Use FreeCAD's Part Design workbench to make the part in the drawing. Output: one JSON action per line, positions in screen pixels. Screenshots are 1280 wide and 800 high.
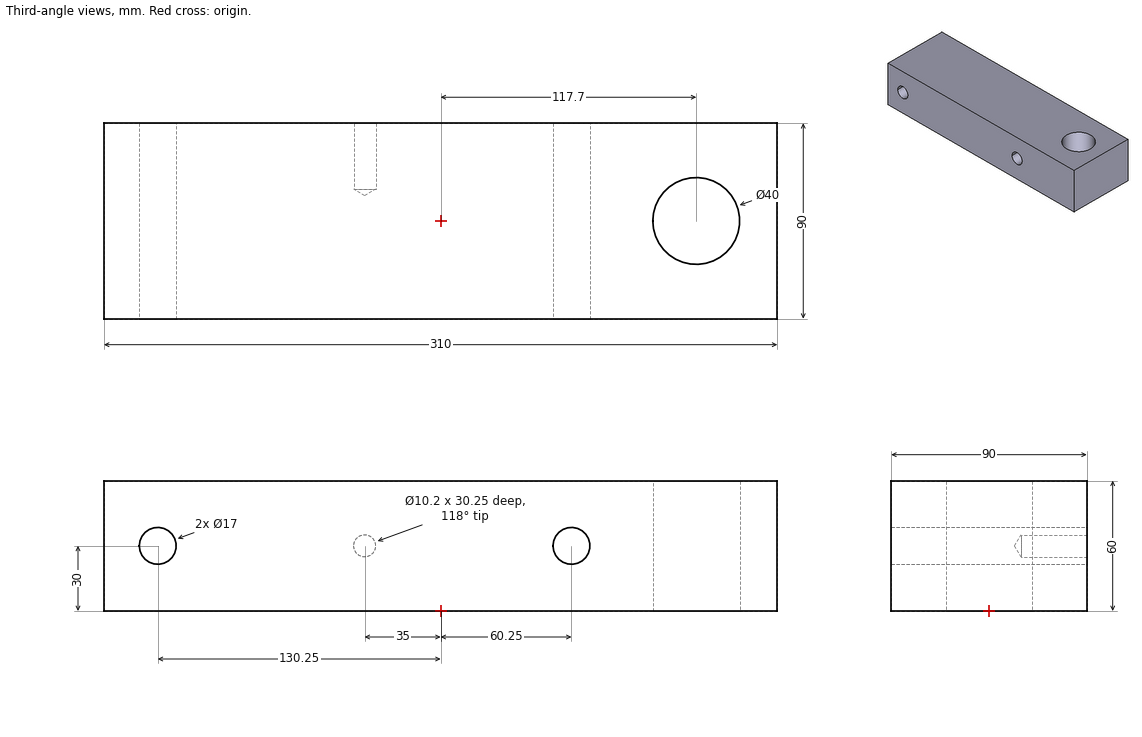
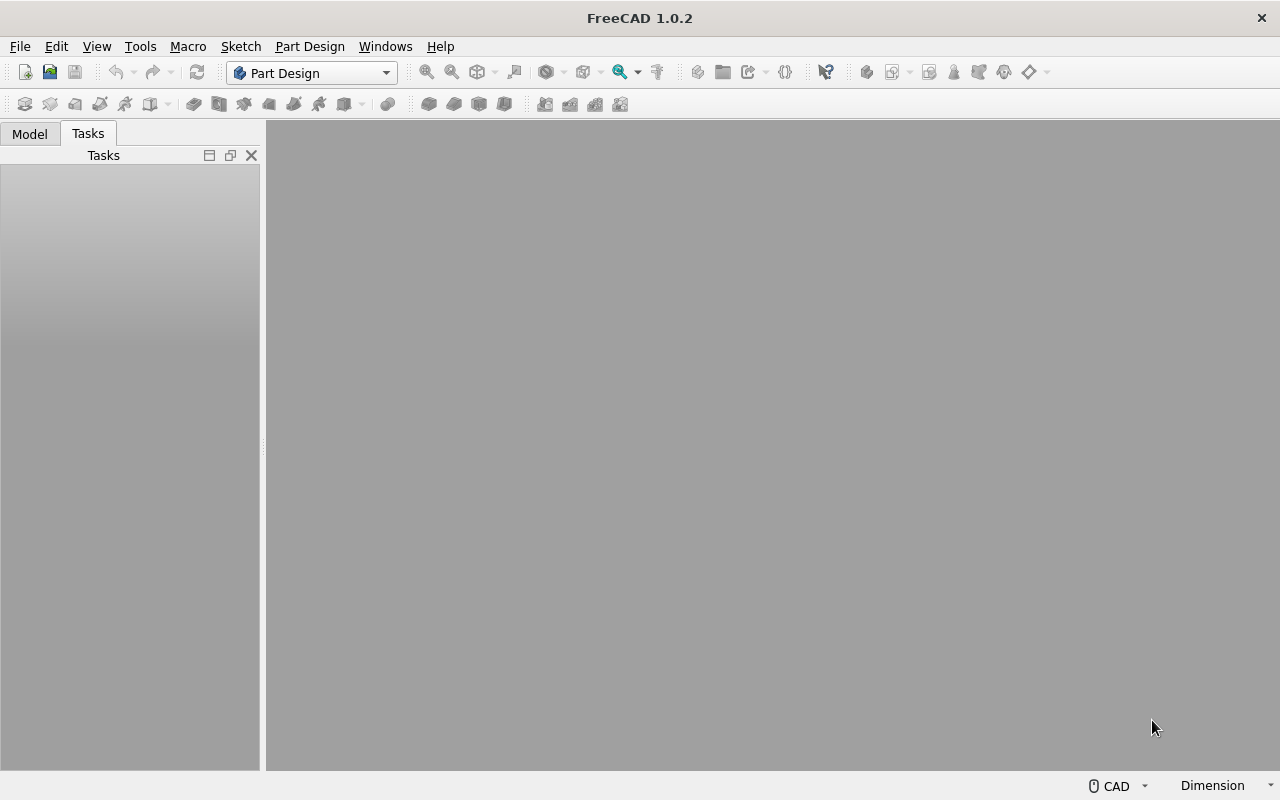
{"action": "left_click", "coordinate": [25, 72]}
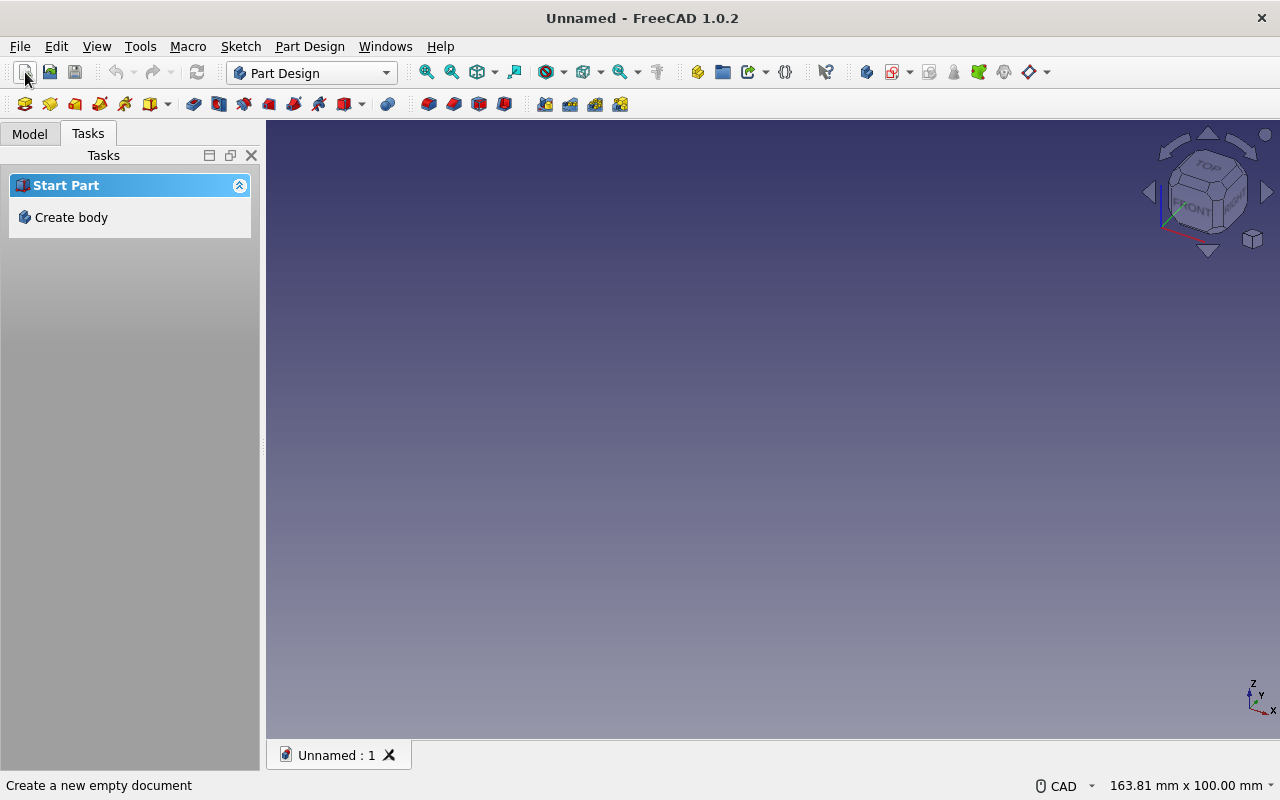
{"action": "left_click", "coordinate": [892, 72]}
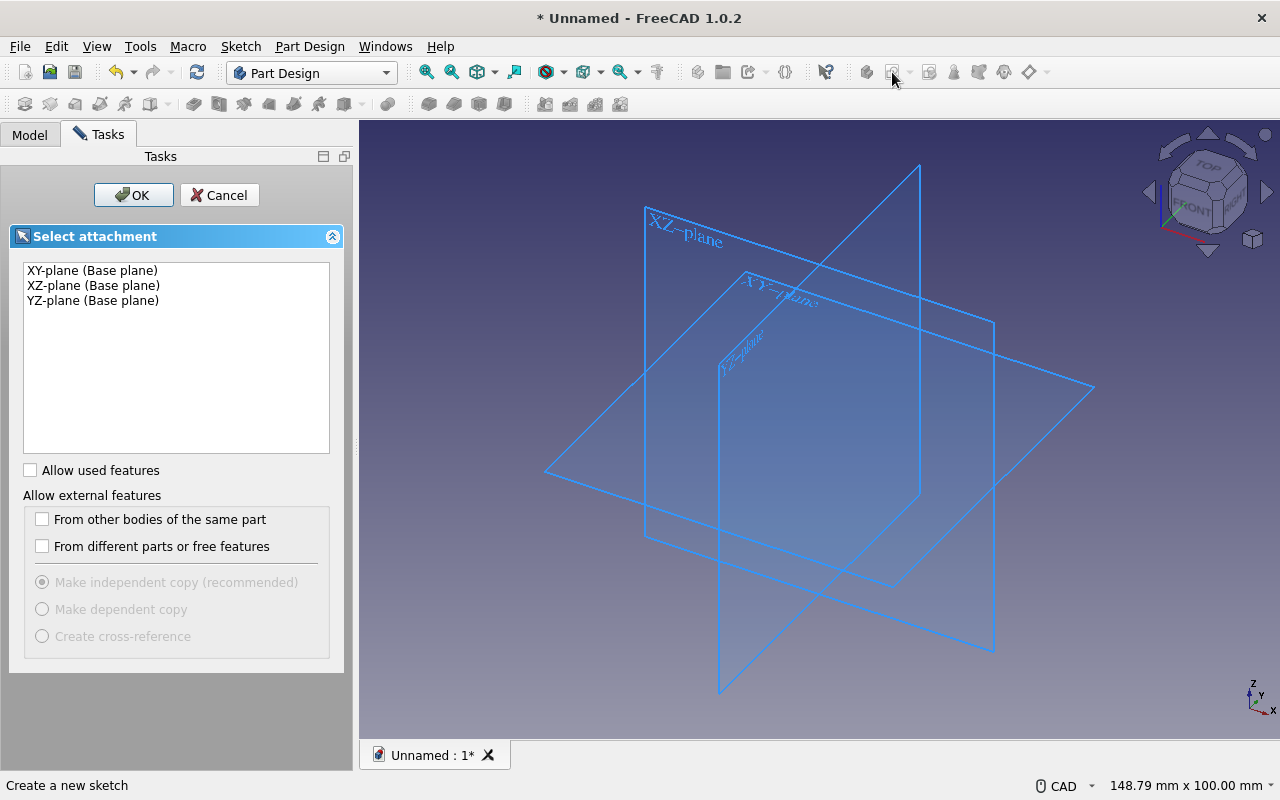
{"action": "left_click", "coordinate": [84, 270]}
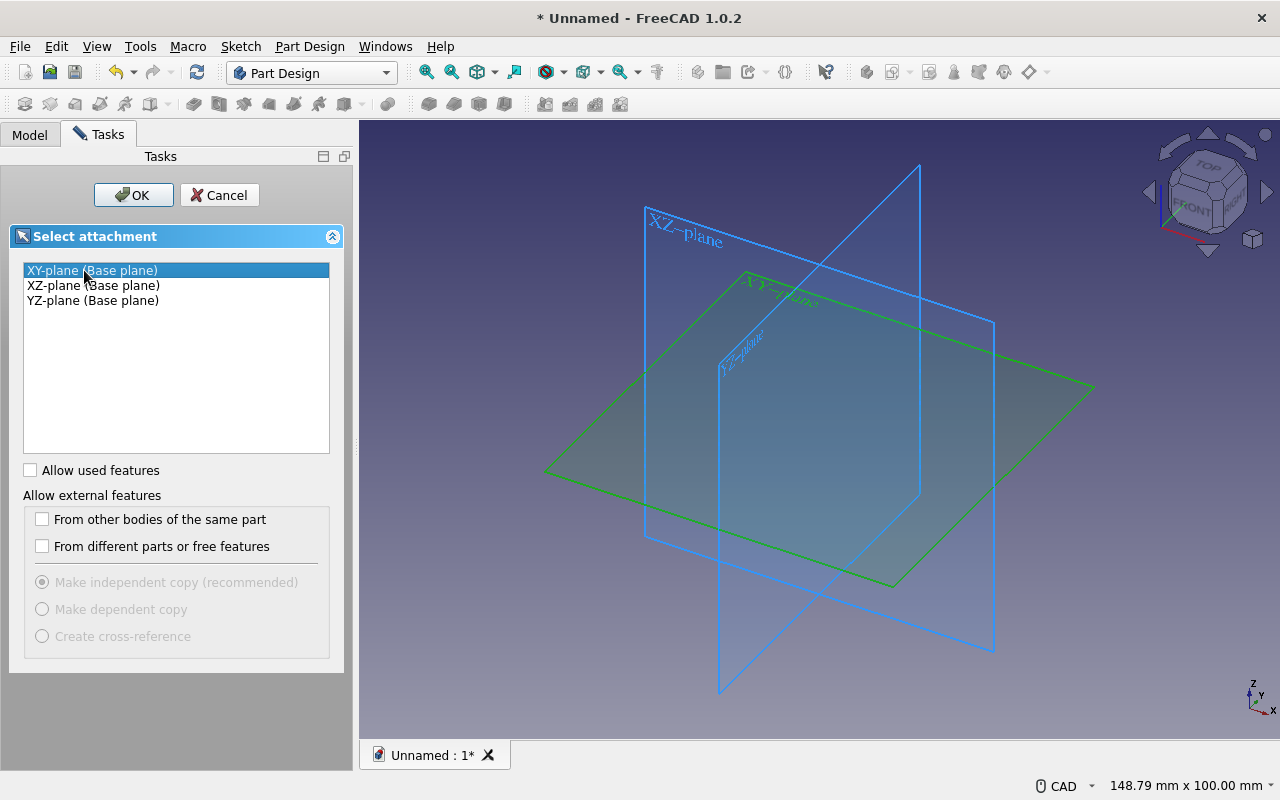
{"action": "left_click", "coordinate": [134, 195]}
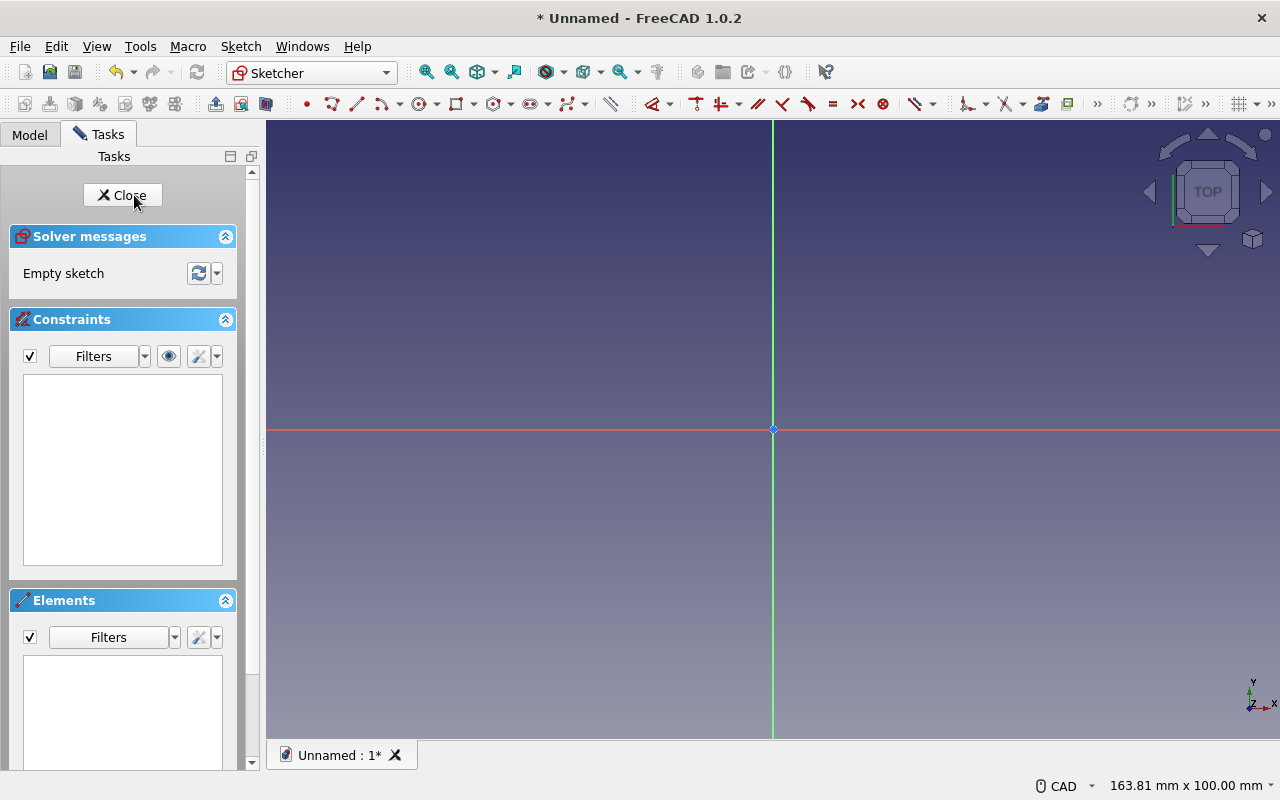
{"action": "scroll", "coordinate": [675, 429], "scroll_direction": "down", "scroll_amount": 6}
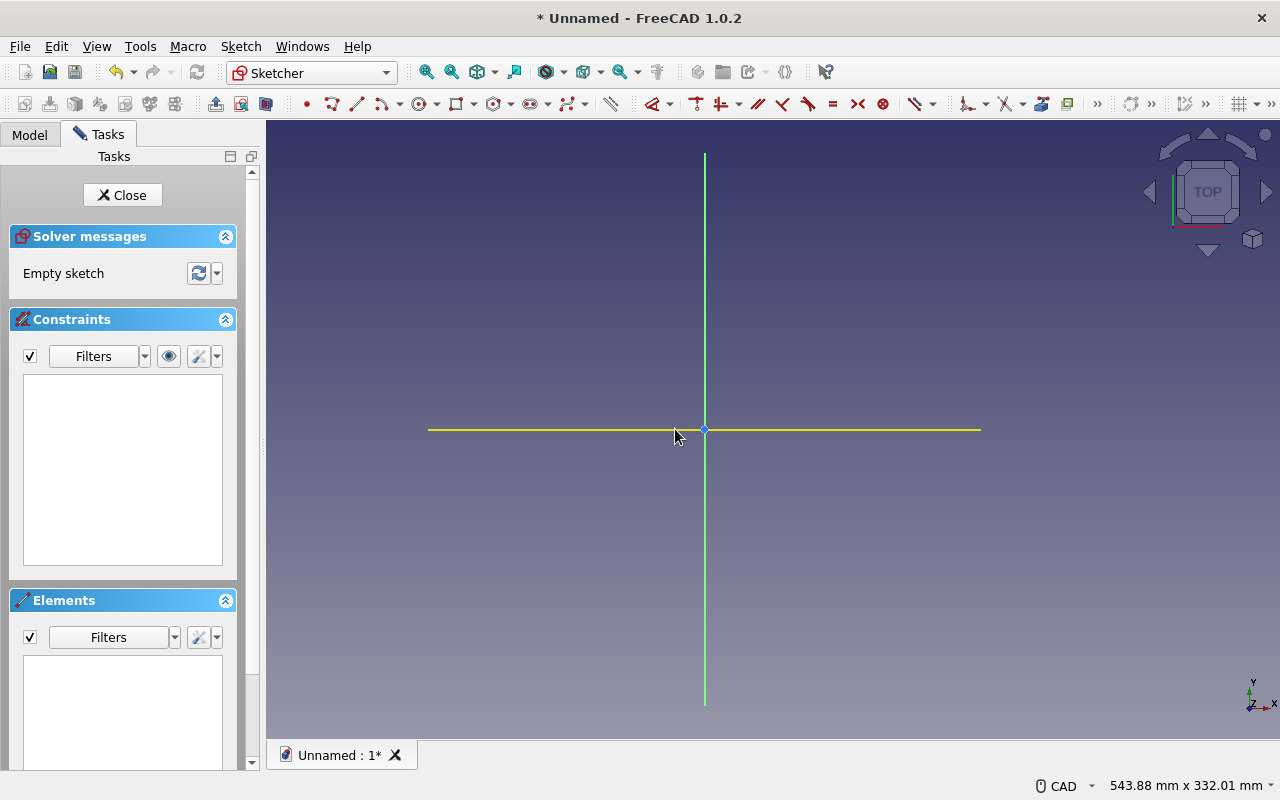
{"action": "key", "text": "g v"}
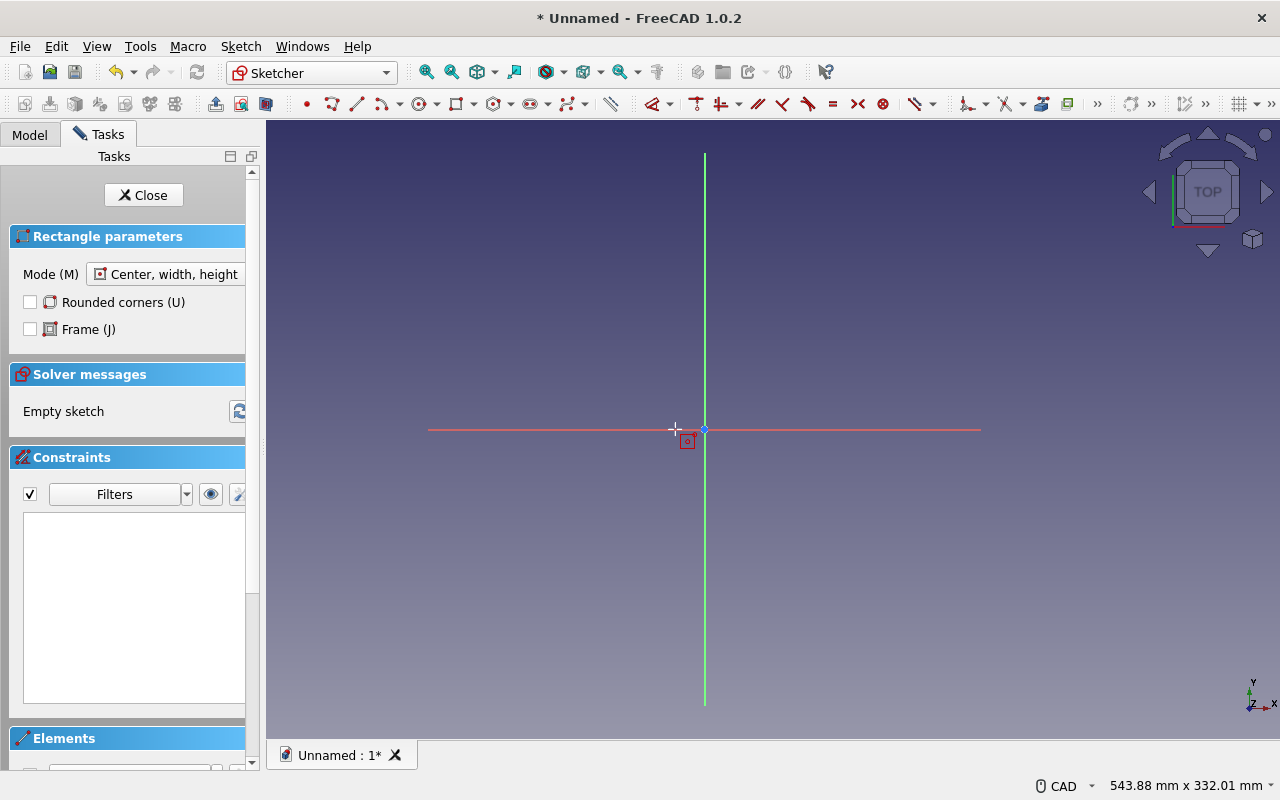
{"action": "left_click", "coordinate": [705, 430]}
{"action": "left_click", "coordinate": [994, 346]}
{"action": "key", "text": "Escape"}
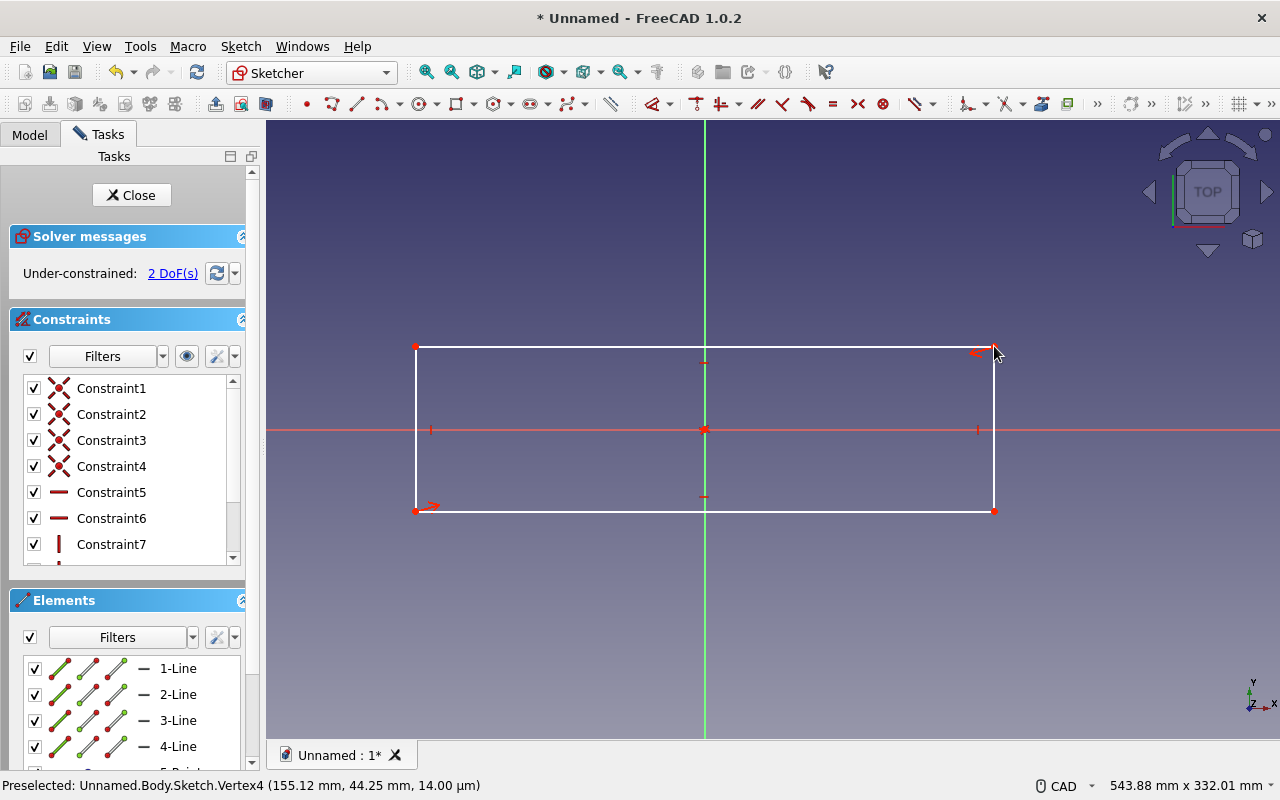
{"action": "left_click", "coordinate": [994, 463]}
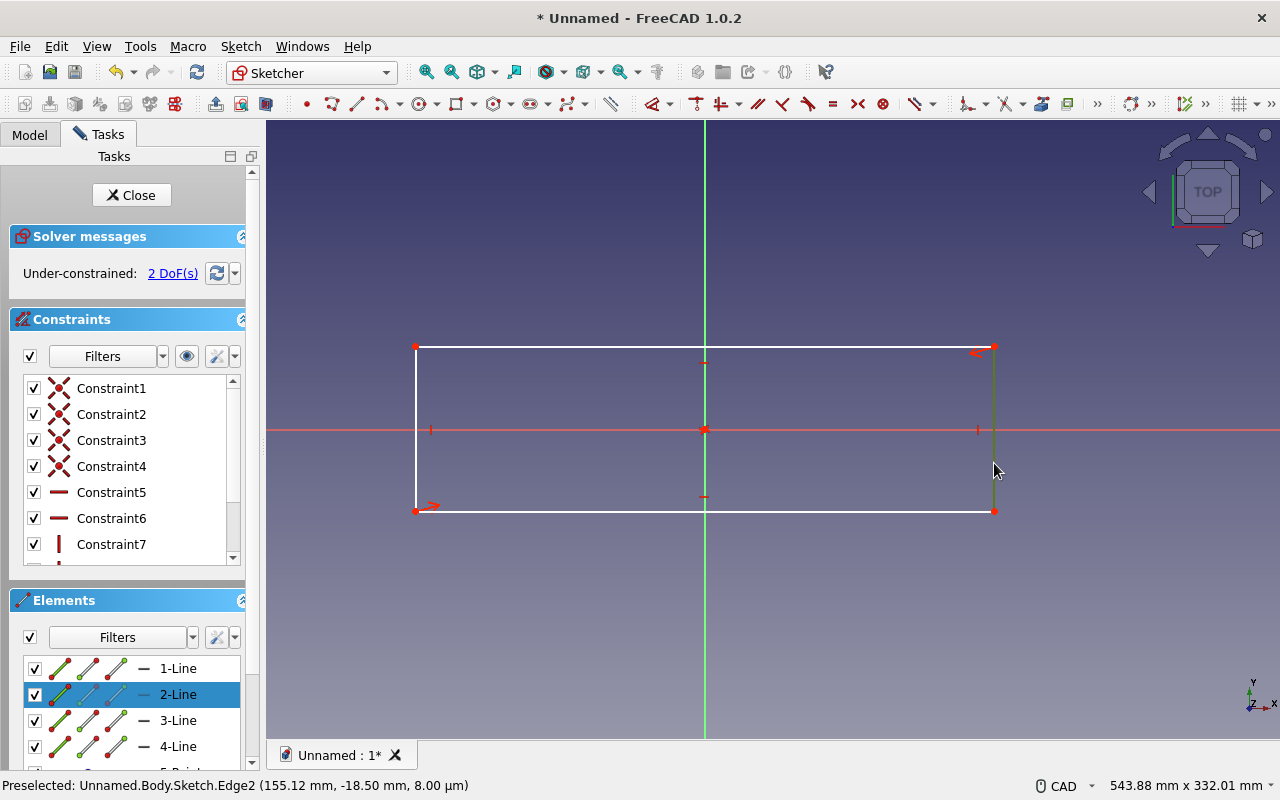
{"action": "key", "text": "i"}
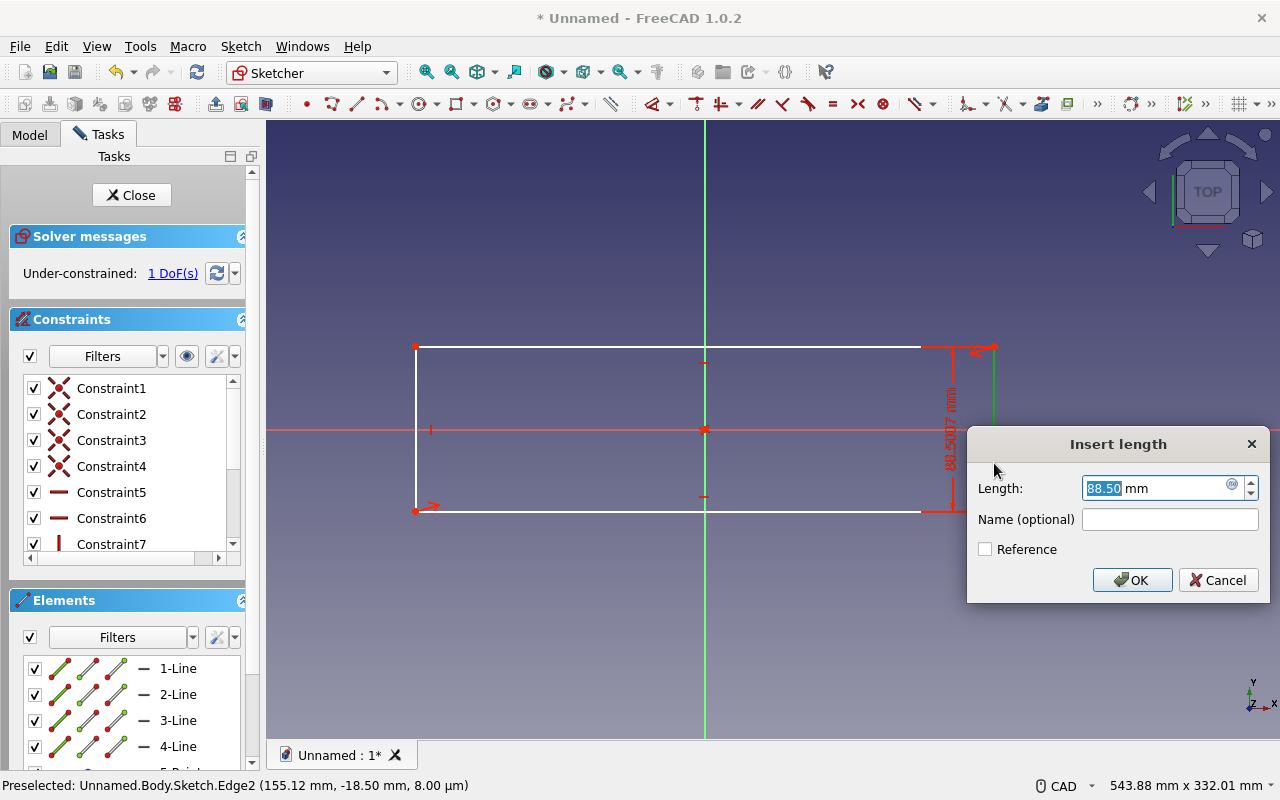
{"action": "type", "text": "90"}
{"action": "key", "text": "Return"}